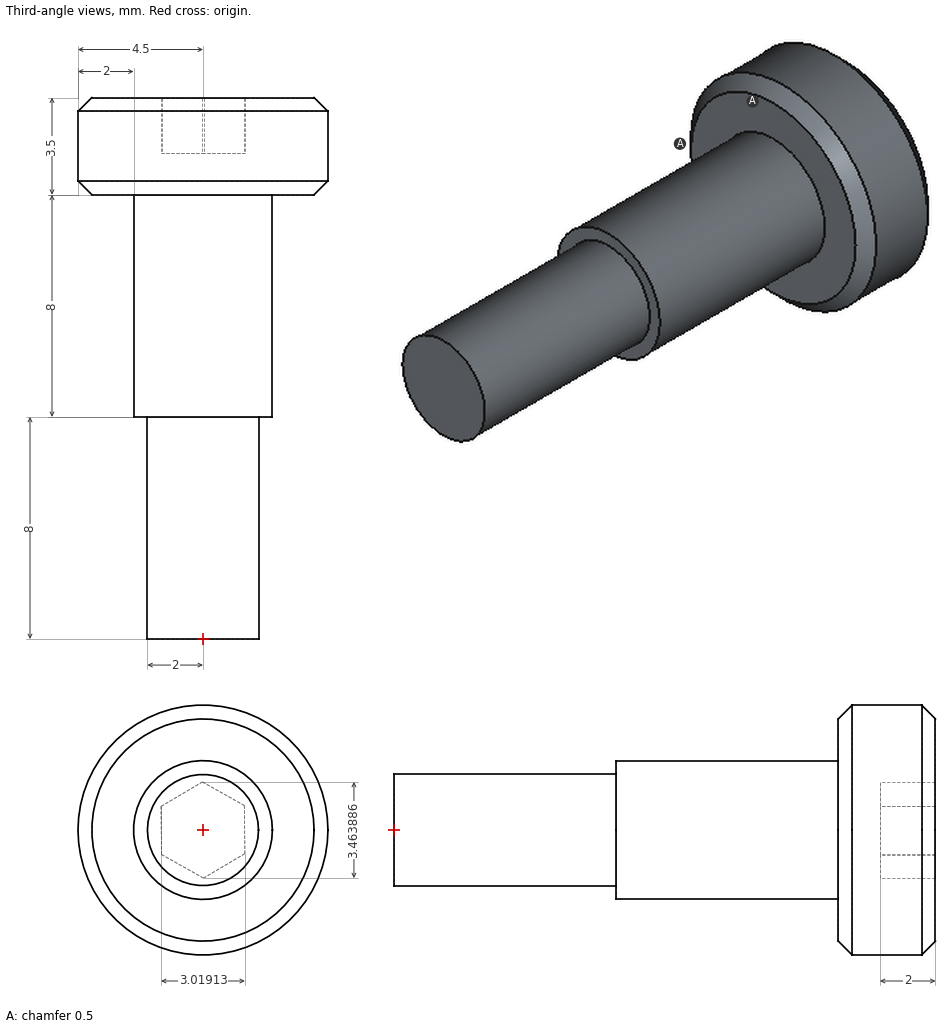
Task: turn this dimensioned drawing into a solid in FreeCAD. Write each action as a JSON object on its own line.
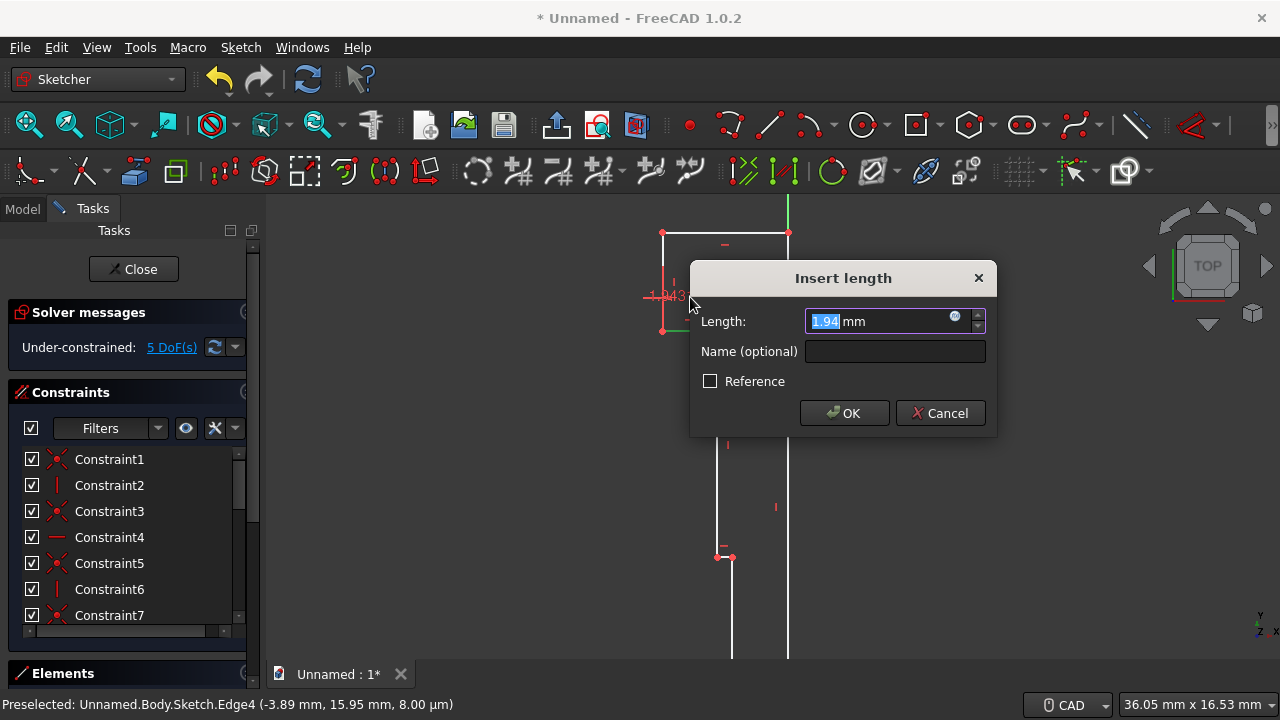
{"action": "type", "text": "2"}
{"action": "key", "text": "Return"}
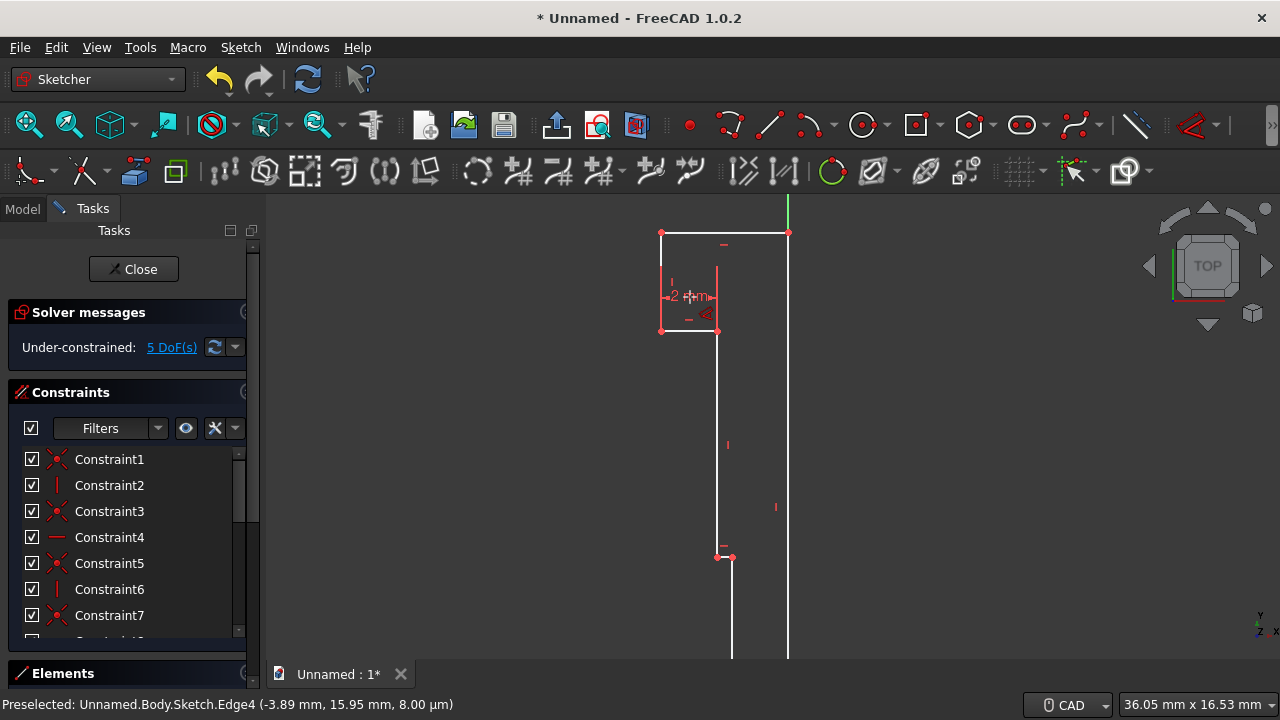
{"action": "left_click", "coordinate": [717, 399]}
{"action": "left_click", "coordinate": [683, 444]}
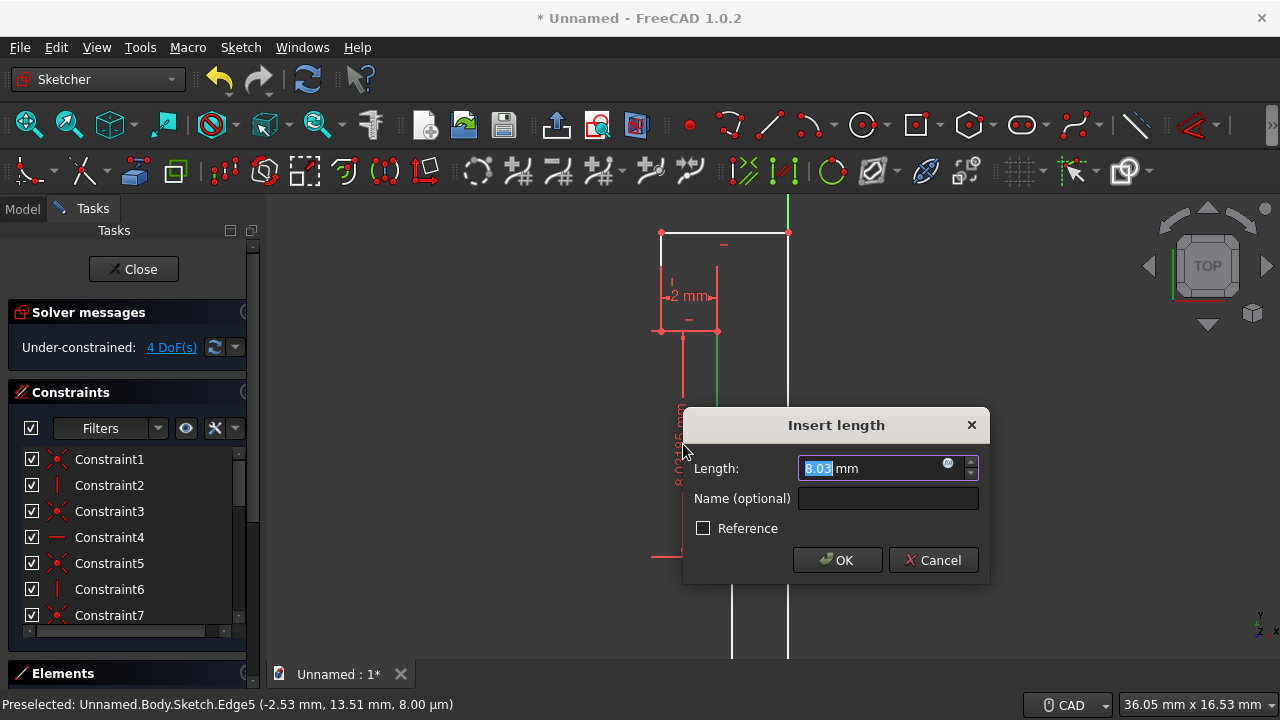
{"action": "type", "text": "8"}
{"action": "key", "text": "Return"}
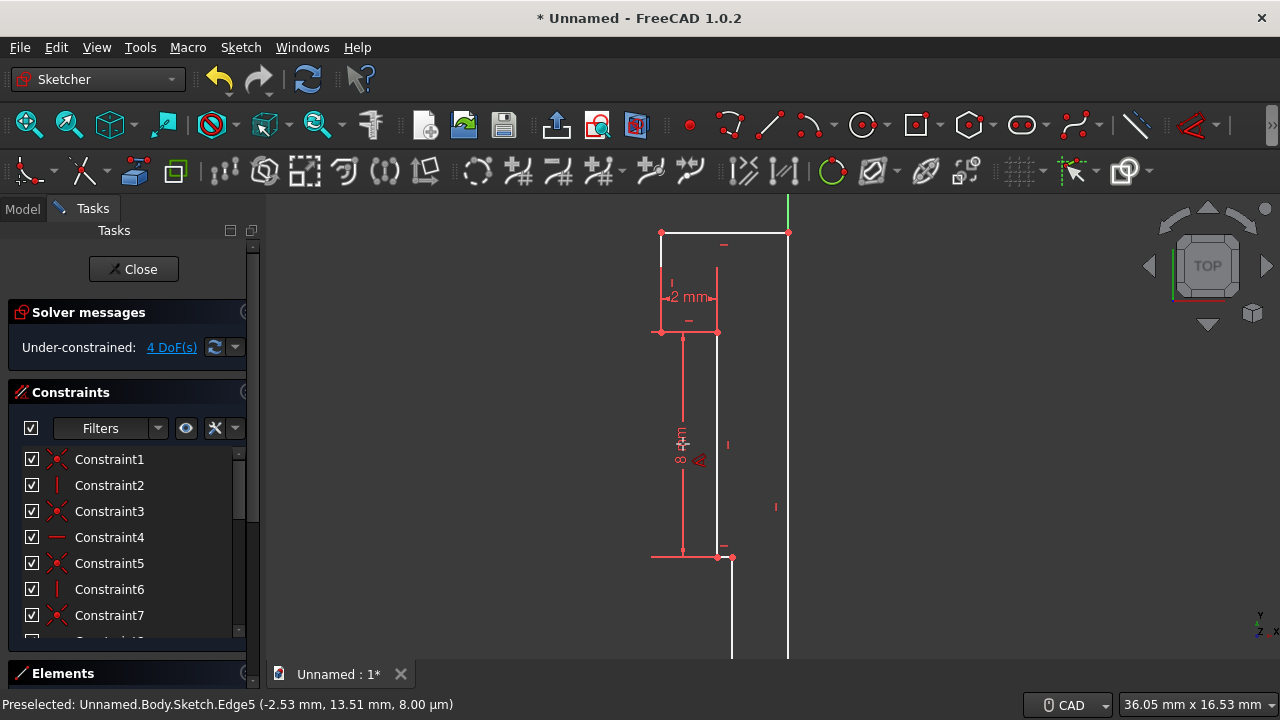
{"action": "left_click", "coordinate": [732, 624]}
{"action": "left_click", "coordinate": [766, 594]}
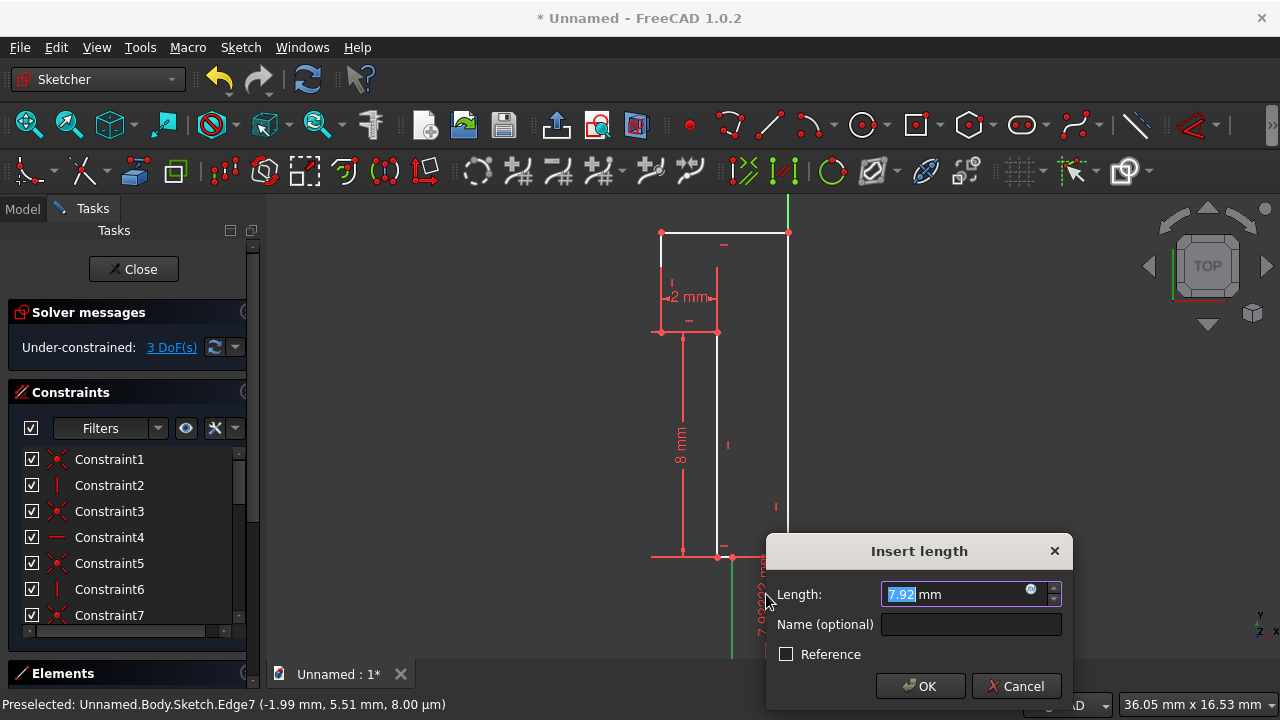
{"action": "type", "text": "8"}
{"action": "key", "text": "Return"}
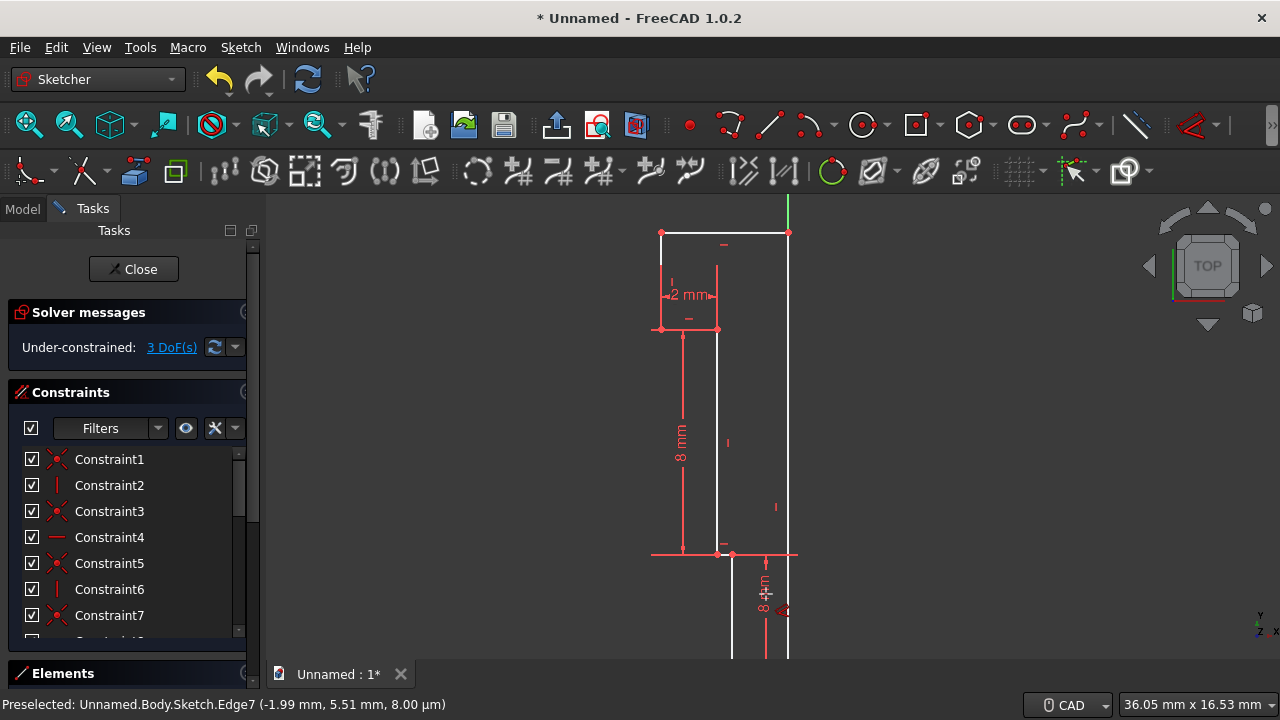
{"action": "scroll", "coordinate": [679, 330], "scroll_direction": "down", "scroll_amount": 3}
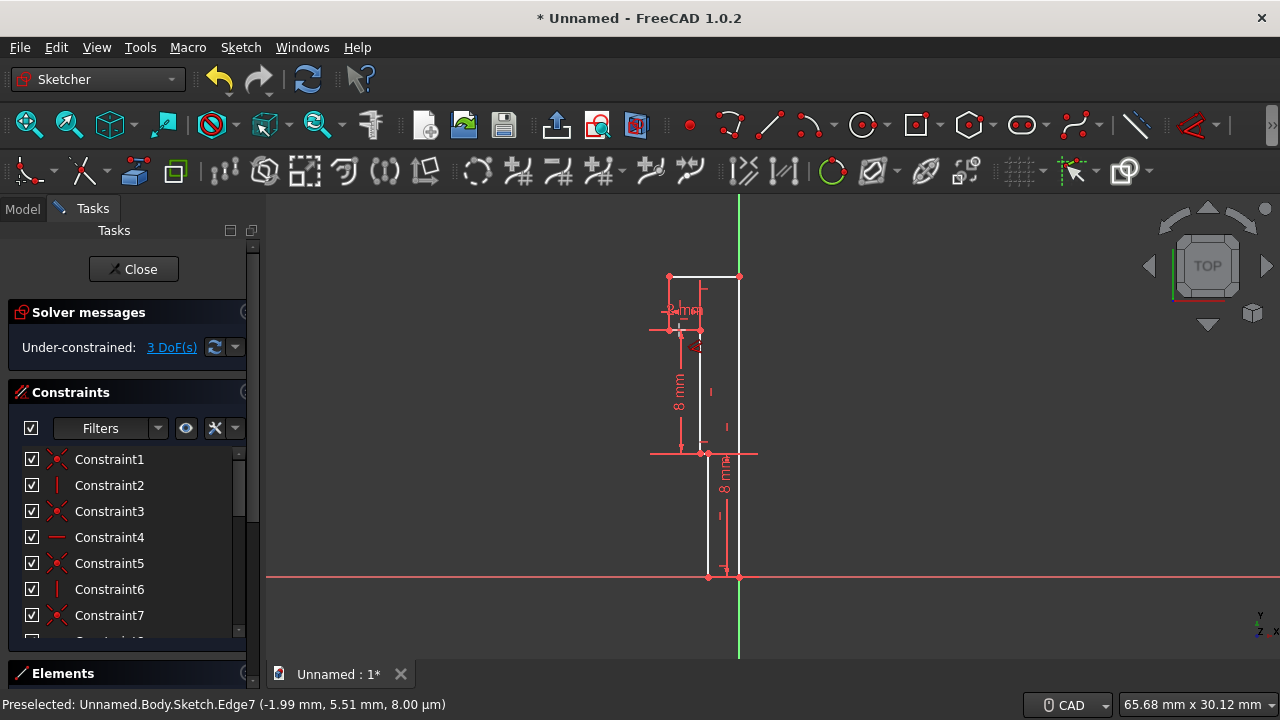
{"action": "scroll", "coordinate": [718, 577], "scroll_direction": "up", "scroll_amount": 3}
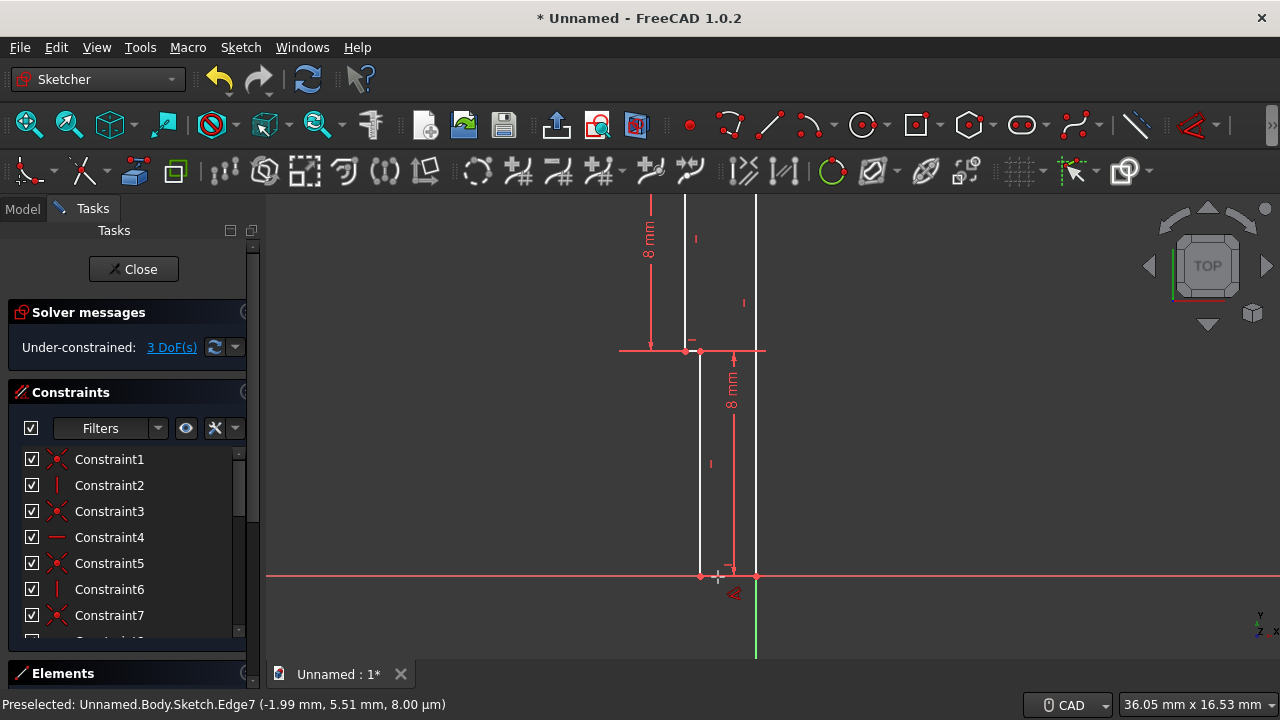
{"action": "left_click", "coordinate": [717, 576]}
{"action": "left_click", "coordinate": [728, 610]}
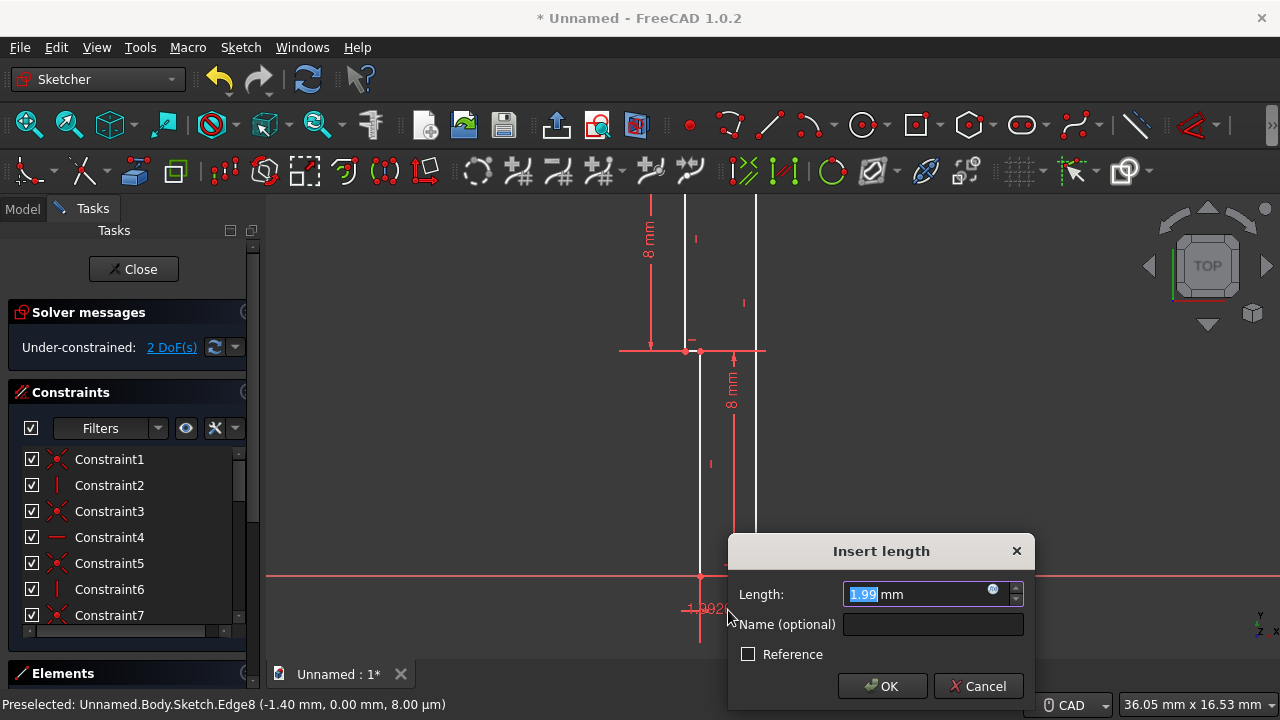
{"action": "type", "text": "2"}
{"action": "key", "text": "Return"}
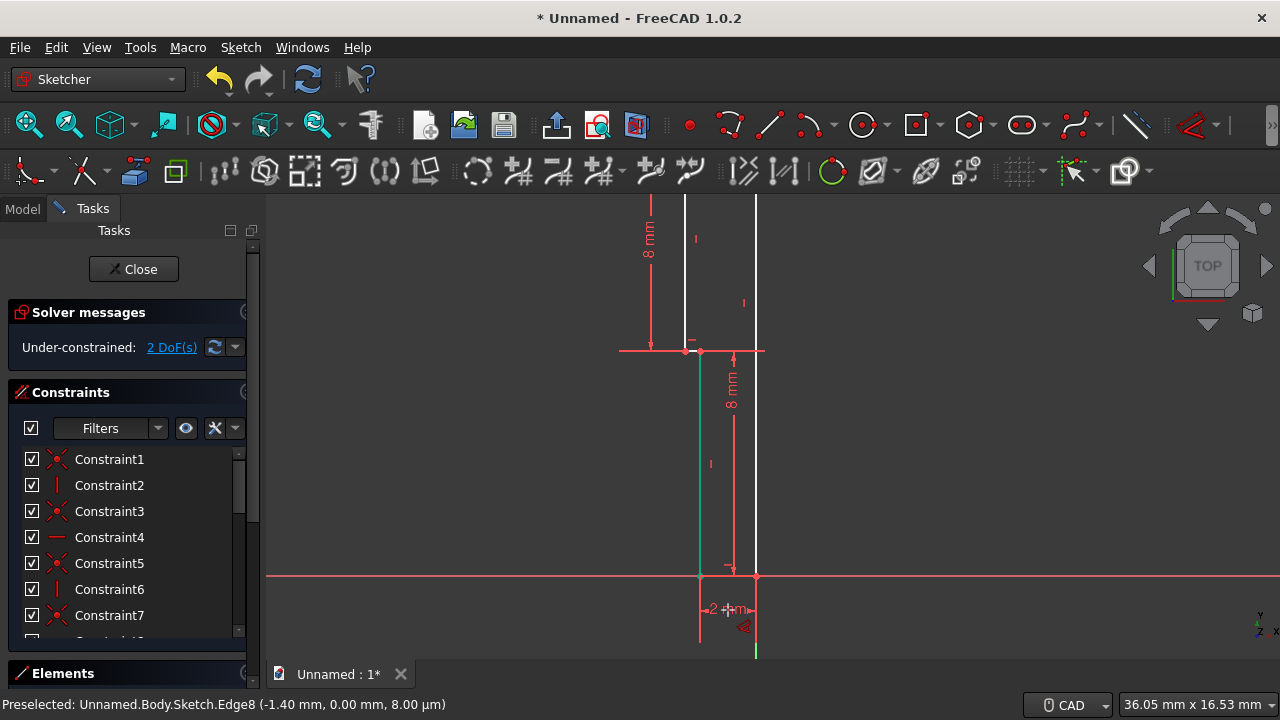
{"action": "scroll", "coordinate": [719, 578], "scroll_direction": "down", "scroll_amount": 3}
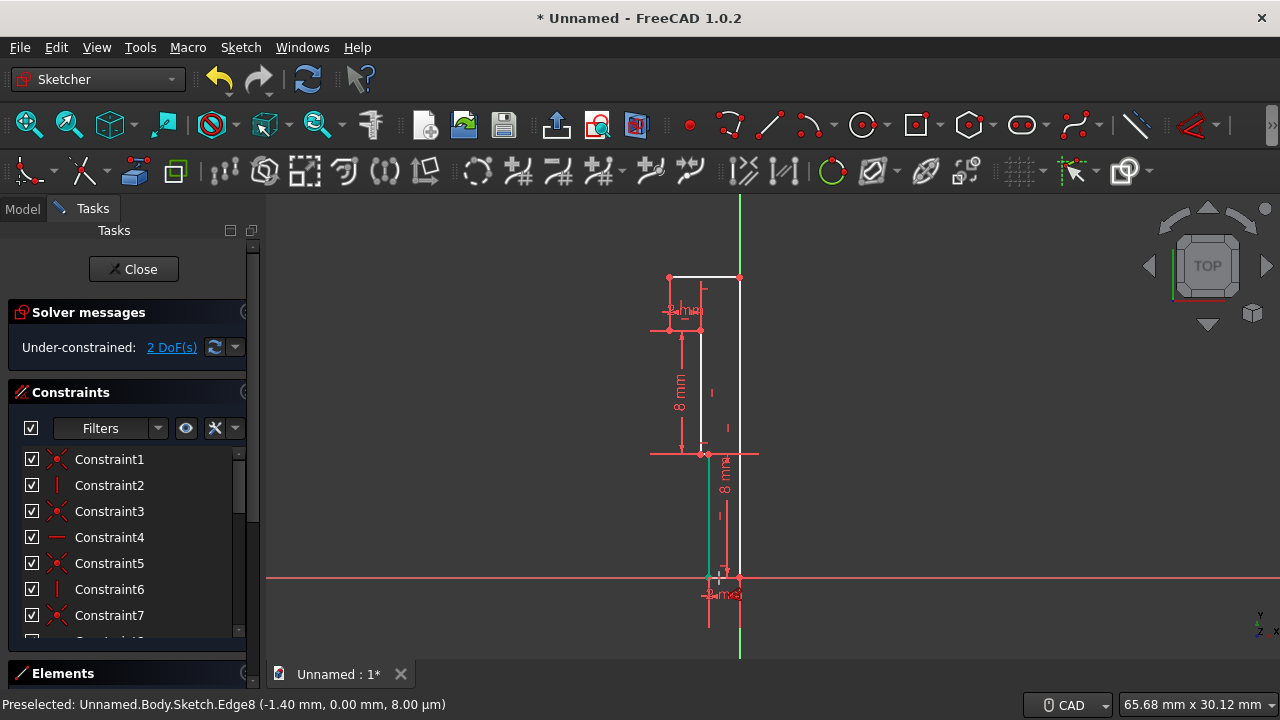
{"action": "left_click", "coordinate": [719, 277]}
{"action": "left_click", "coordinate": [705, 243]}